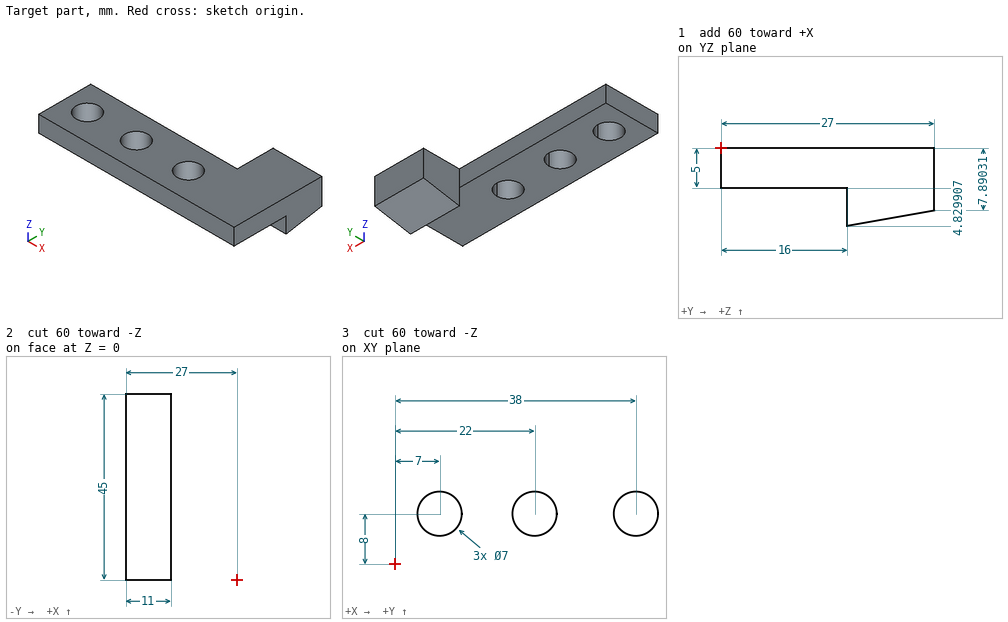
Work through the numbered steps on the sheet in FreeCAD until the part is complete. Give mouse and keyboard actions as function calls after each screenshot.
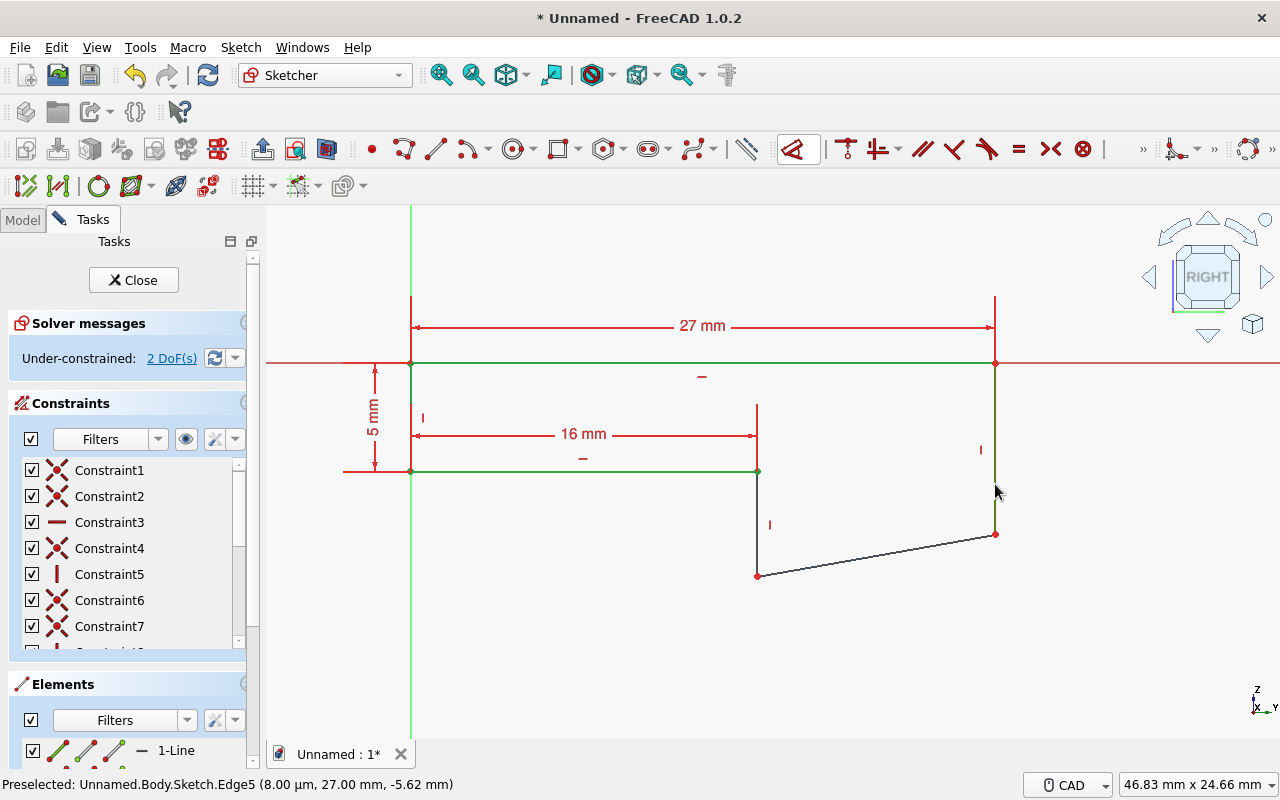
key(i)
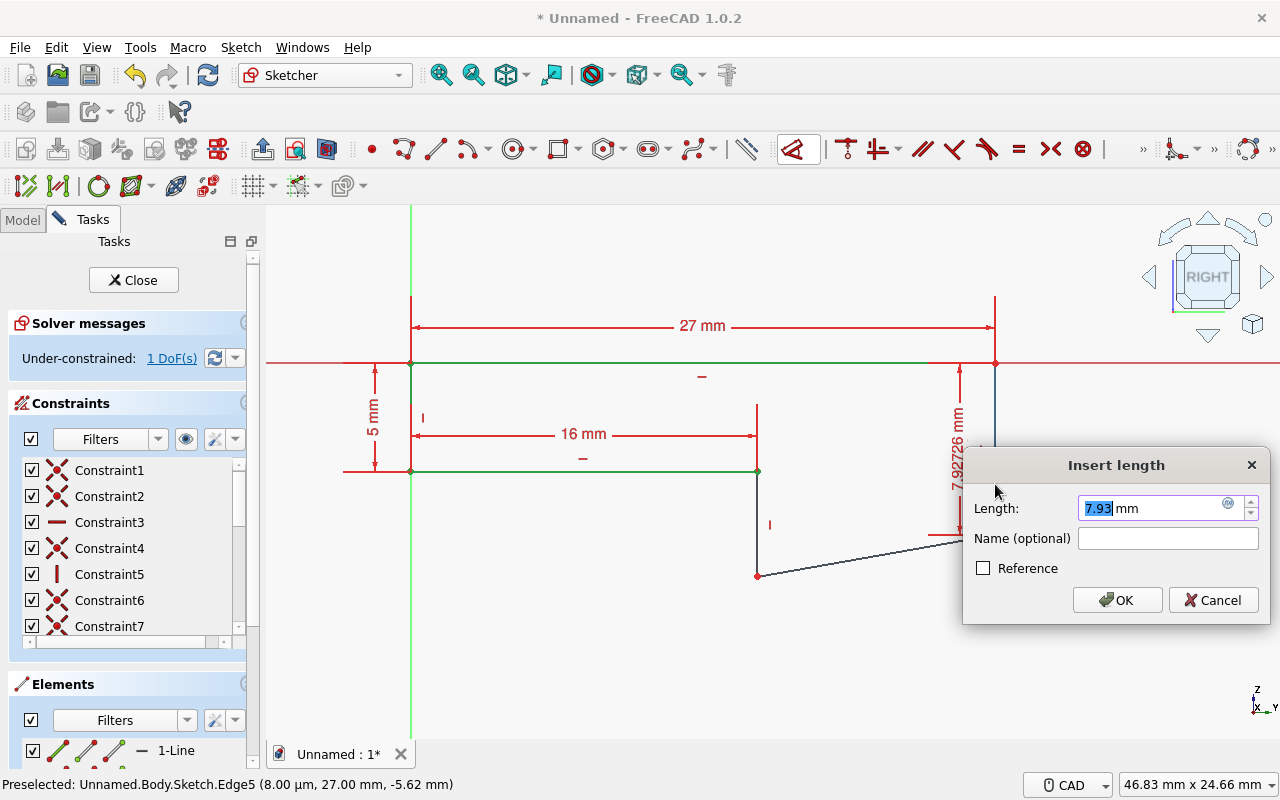
text(7.89031)
key(Return)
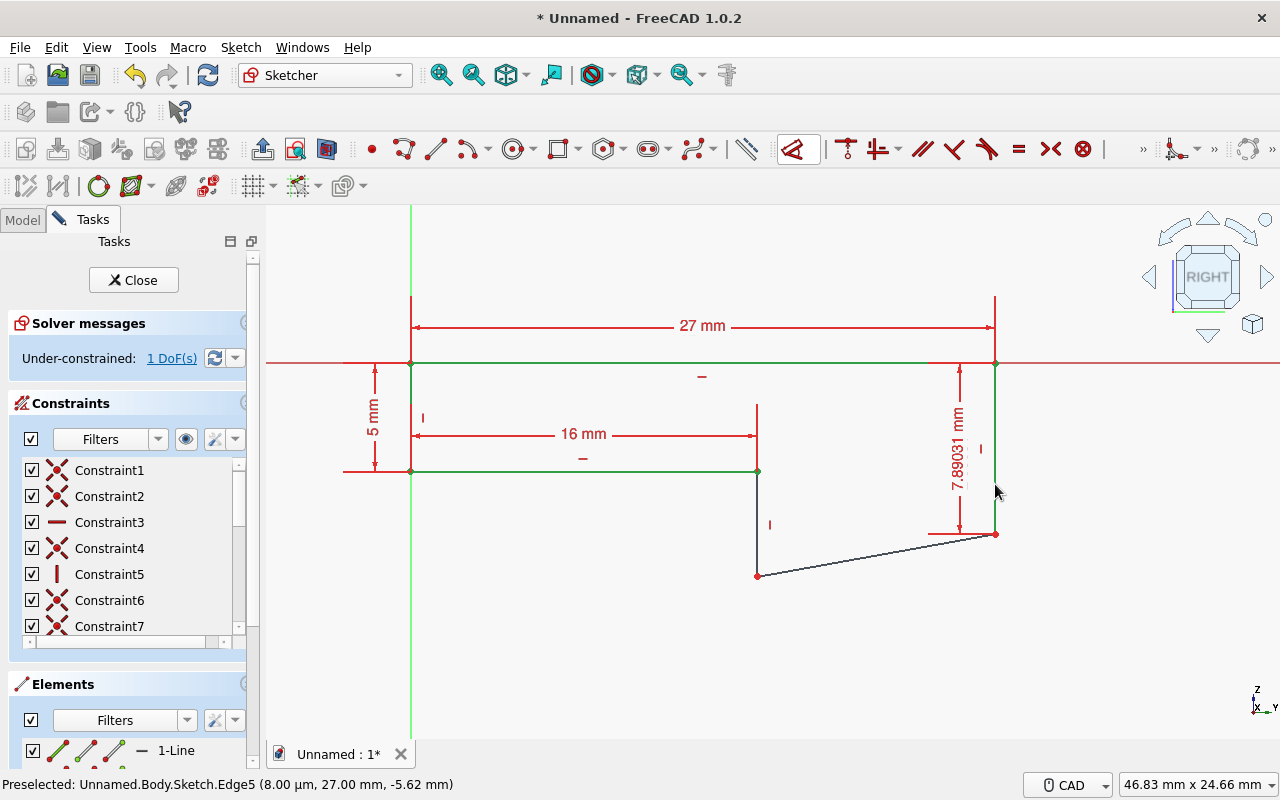
click(757, 503)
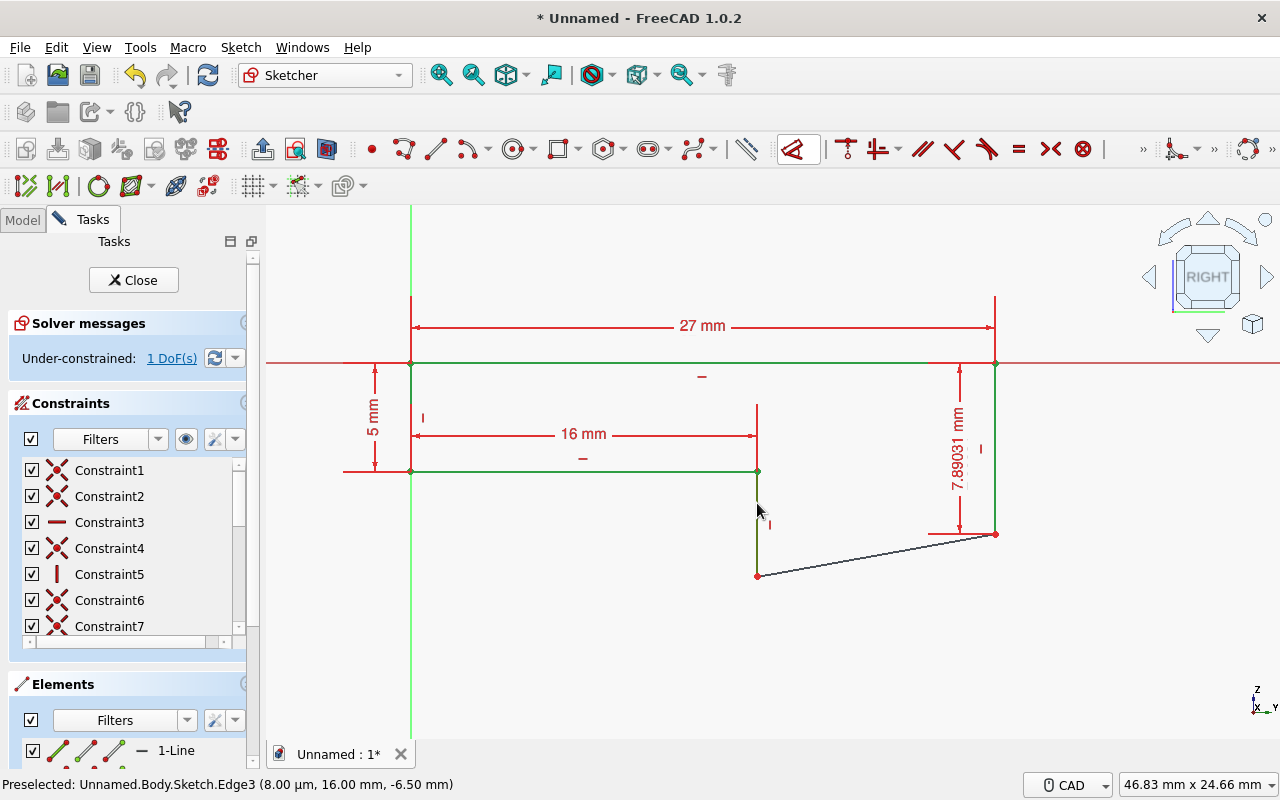
click(814, 150)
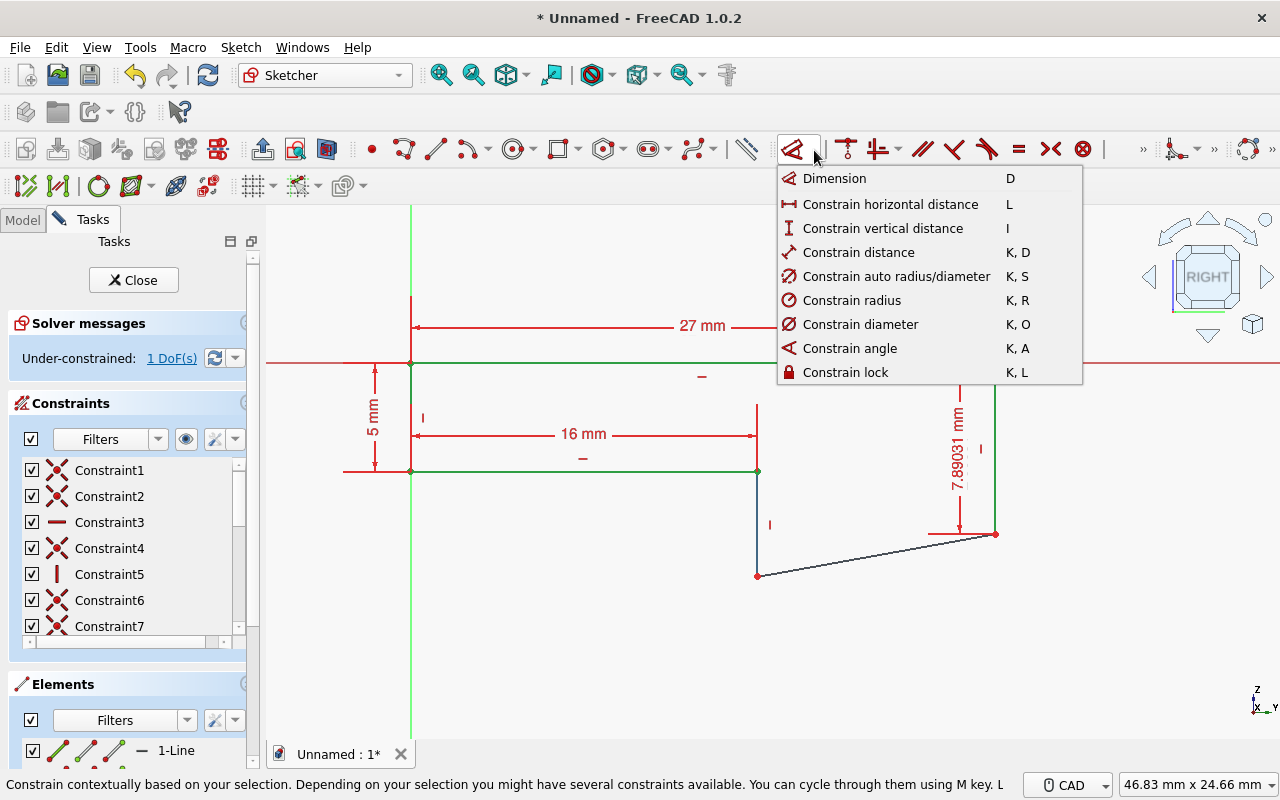
click(930, 228)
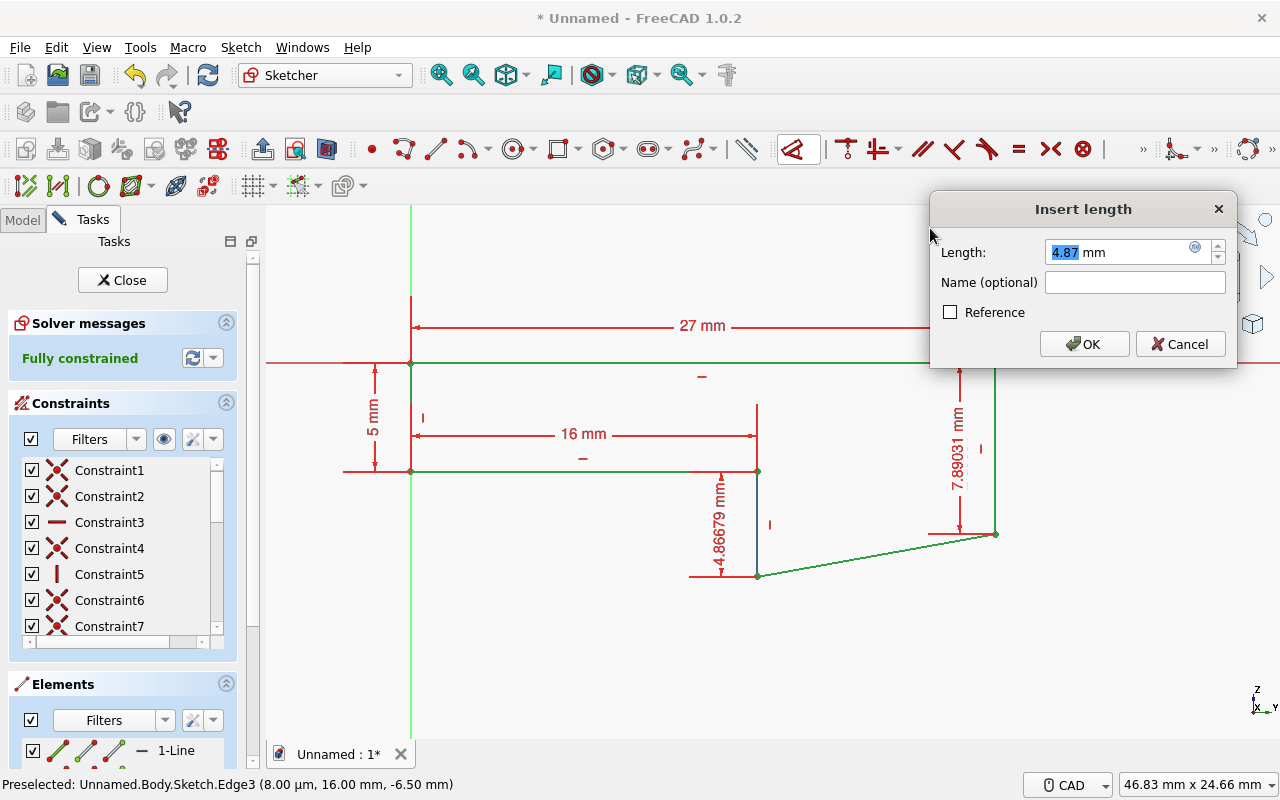
text(4.829907)
key(Return)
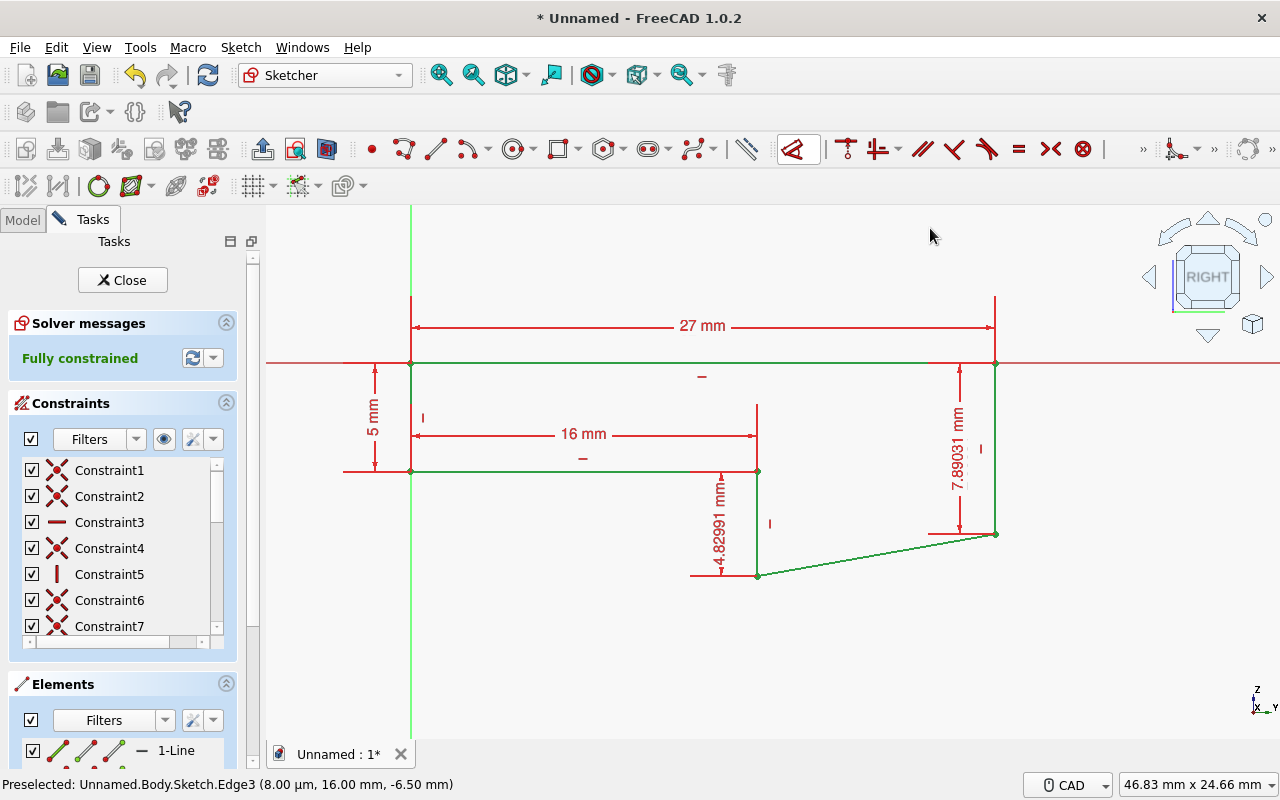
click(123, 280)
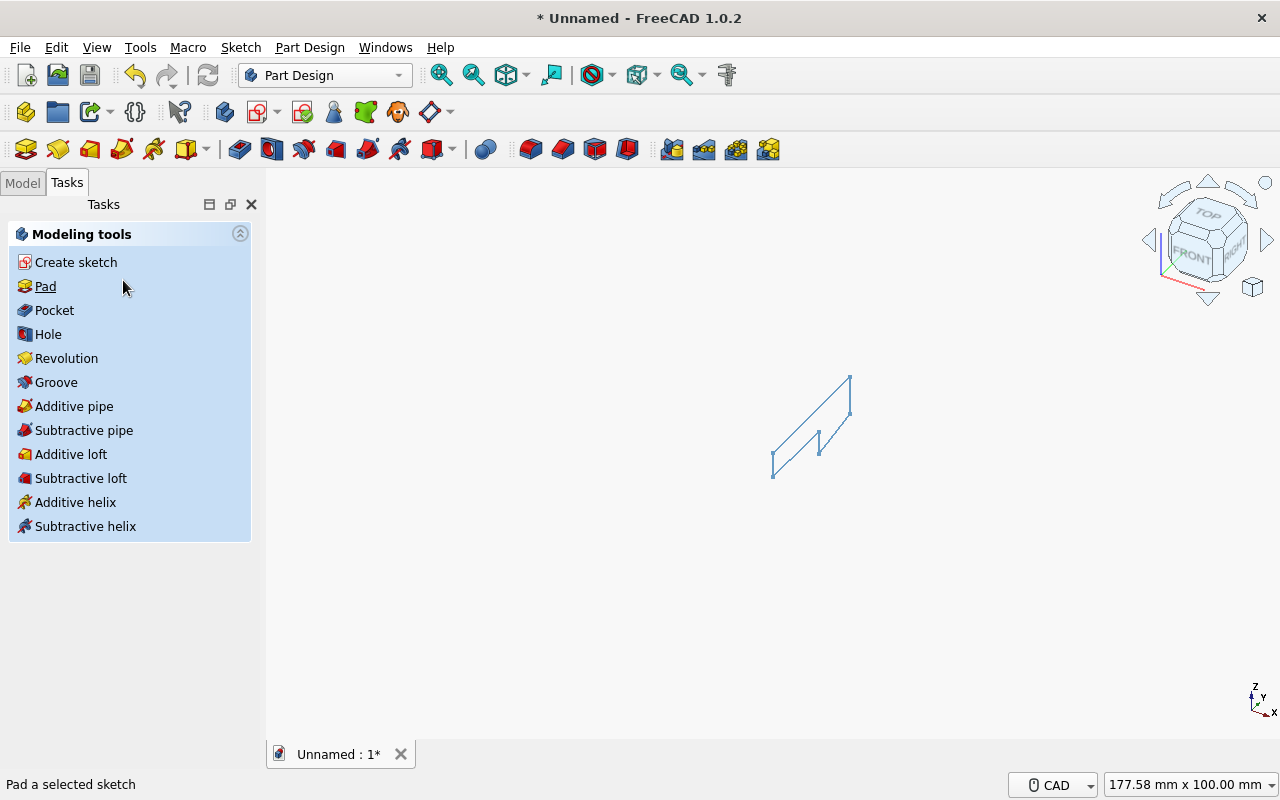
click(26, 150)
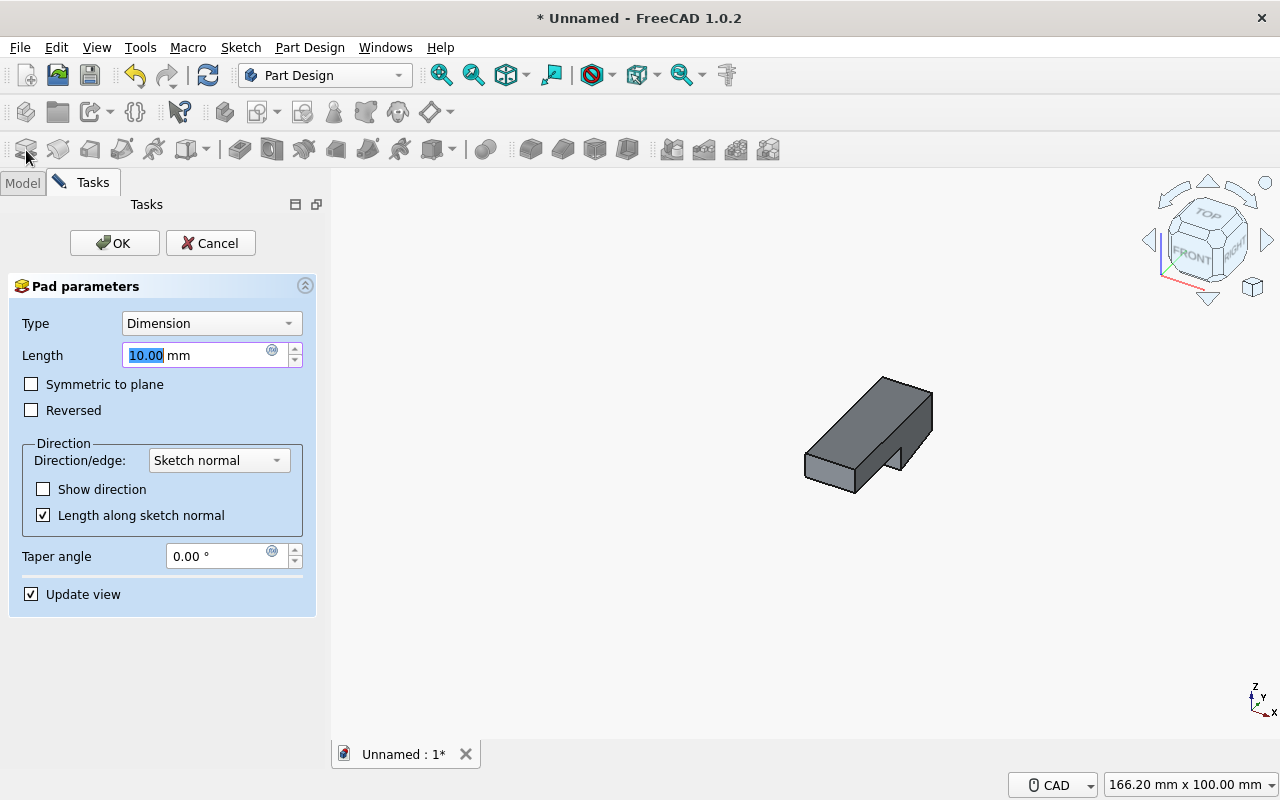
text(60)
key(Tab)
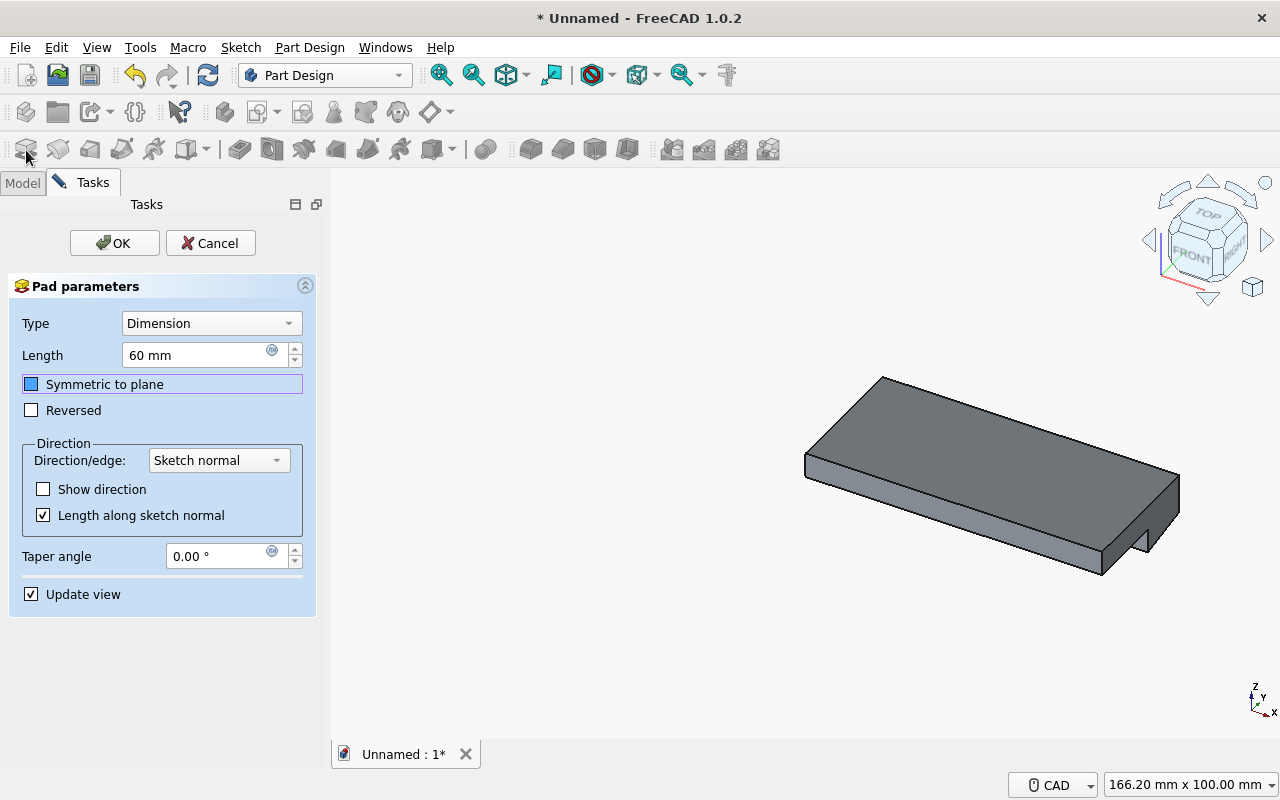
click(115, 243)